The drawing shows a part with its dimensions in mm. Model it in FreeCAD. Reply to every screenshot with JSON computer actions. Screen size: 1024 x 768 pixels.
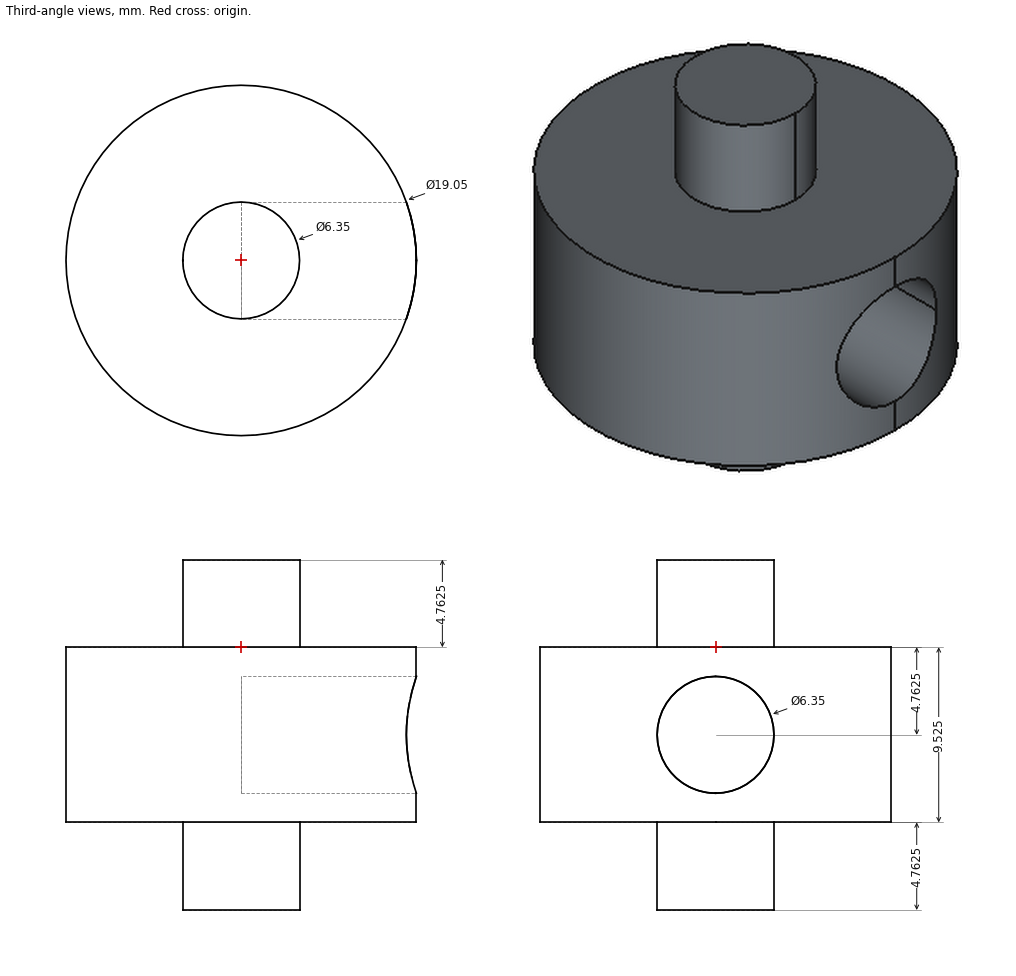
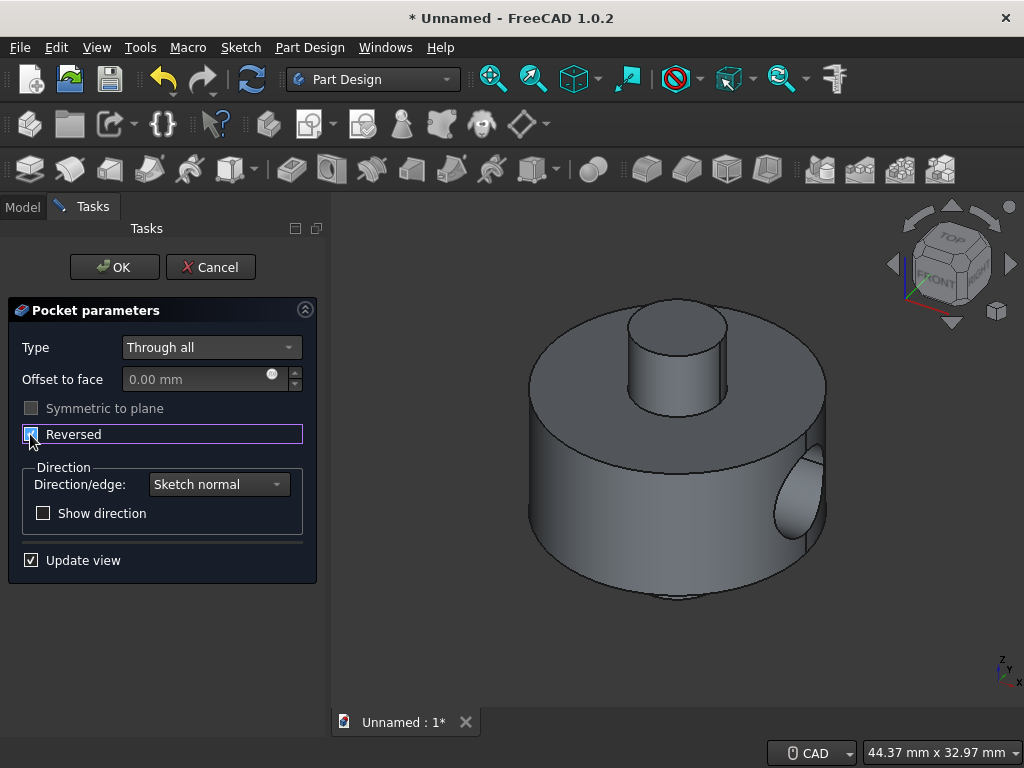
{"action": "left_click", "coordinate": [115, 267]}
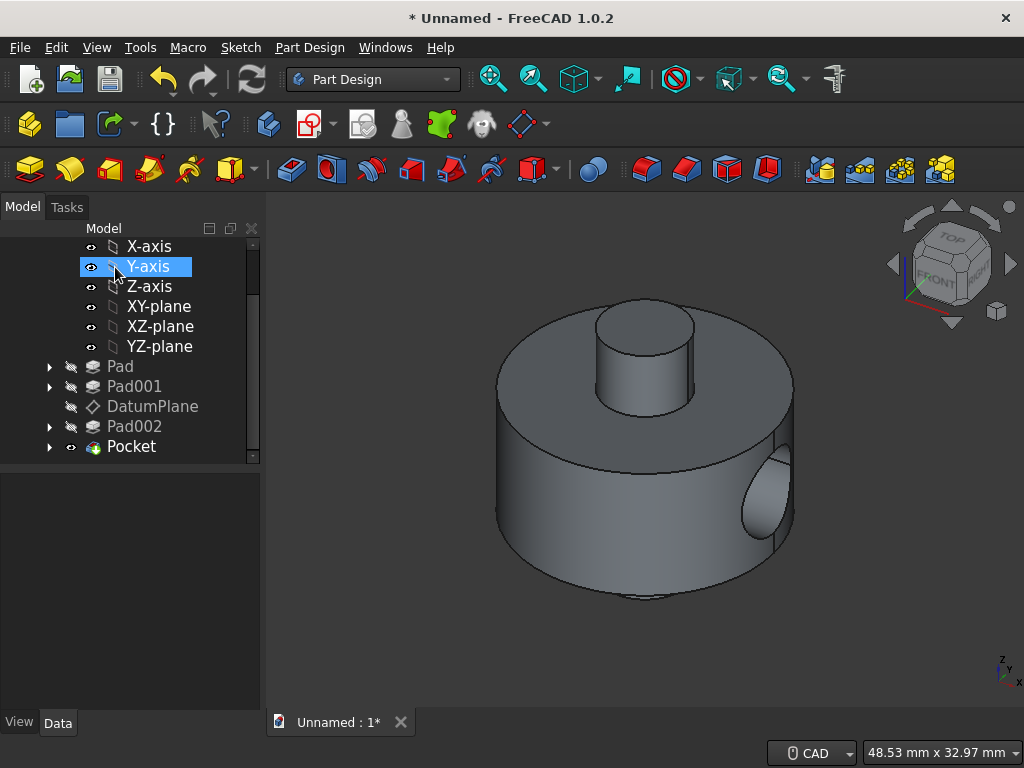
{"action": "key", "text": "0"}